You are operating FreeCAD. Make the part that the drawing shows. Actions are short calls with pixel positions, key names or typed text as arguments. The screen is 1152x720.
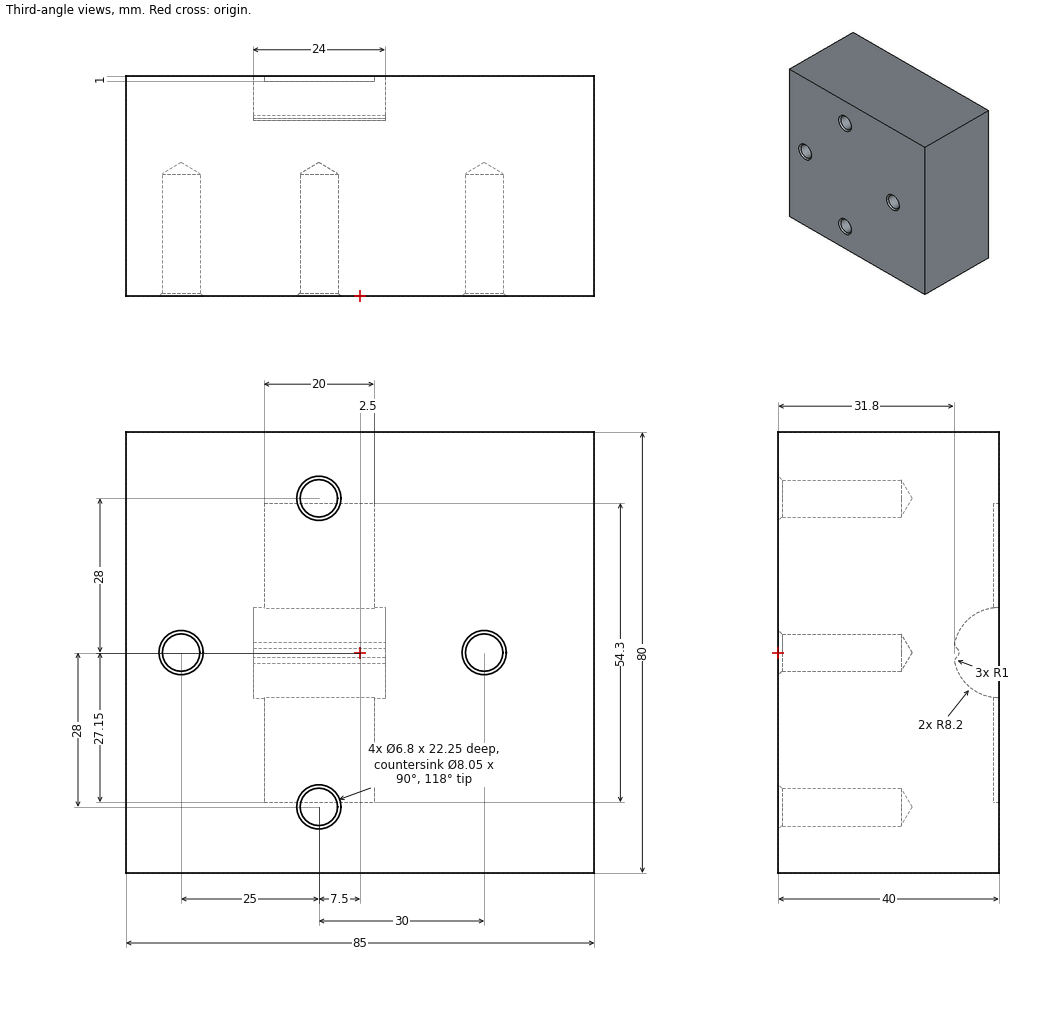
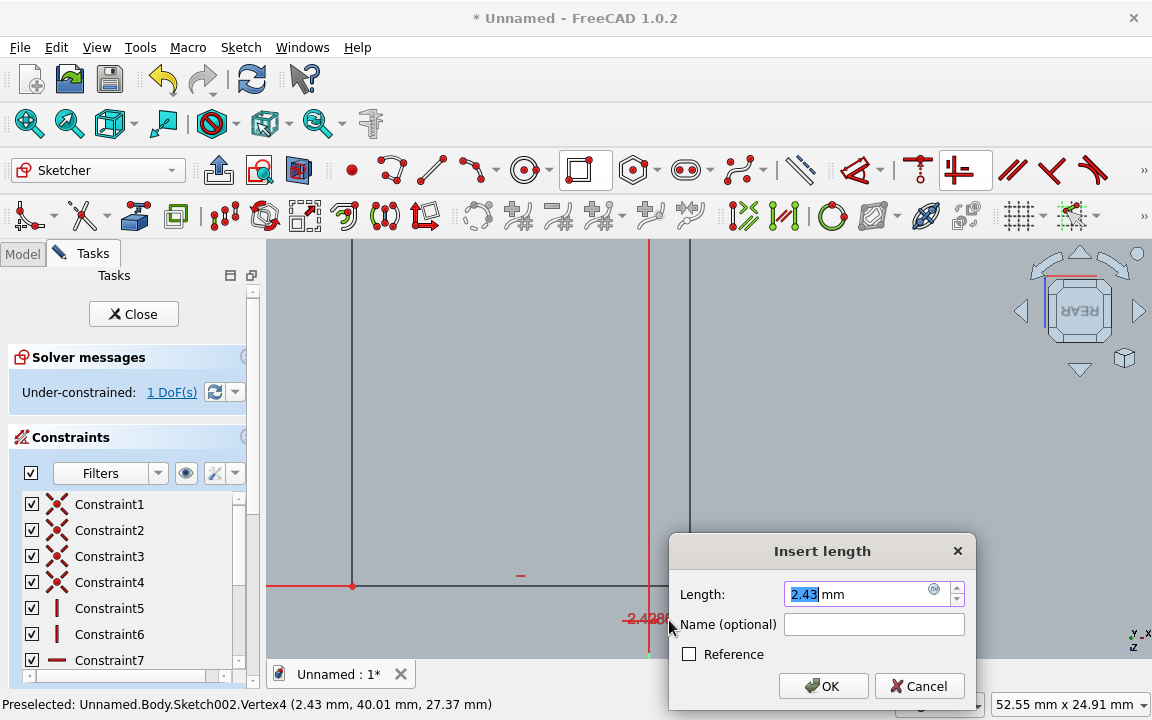
text(2.5)
key(Return)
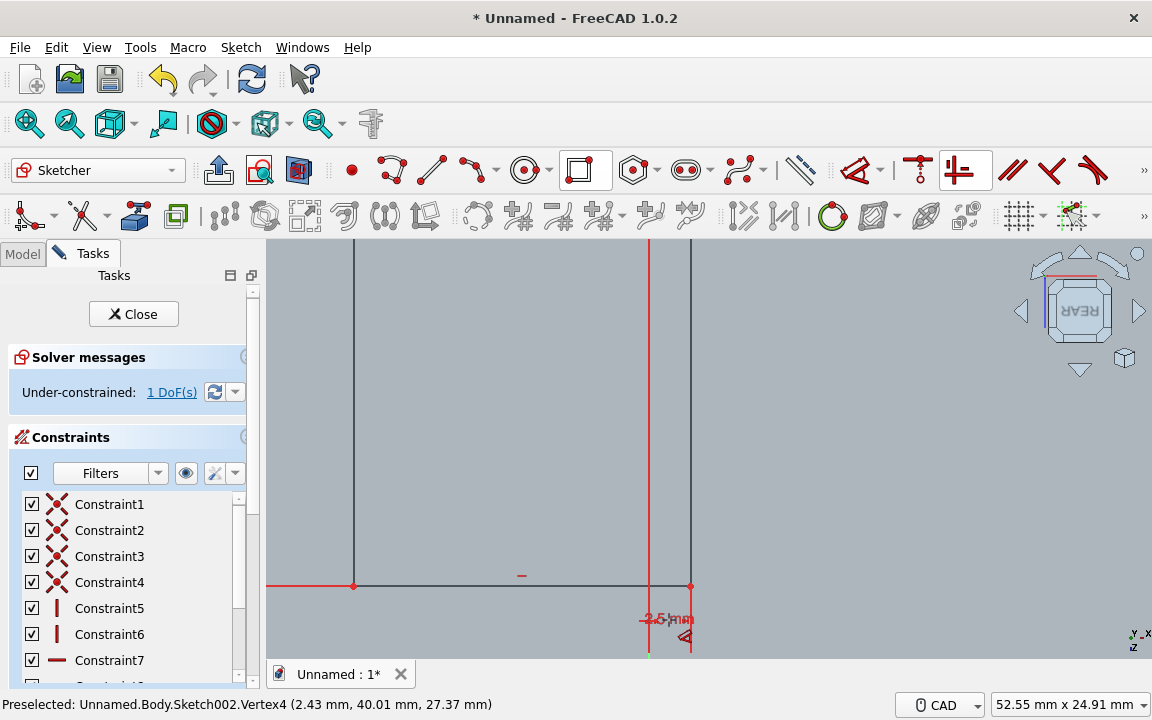
scroll(691, 589, down, 6)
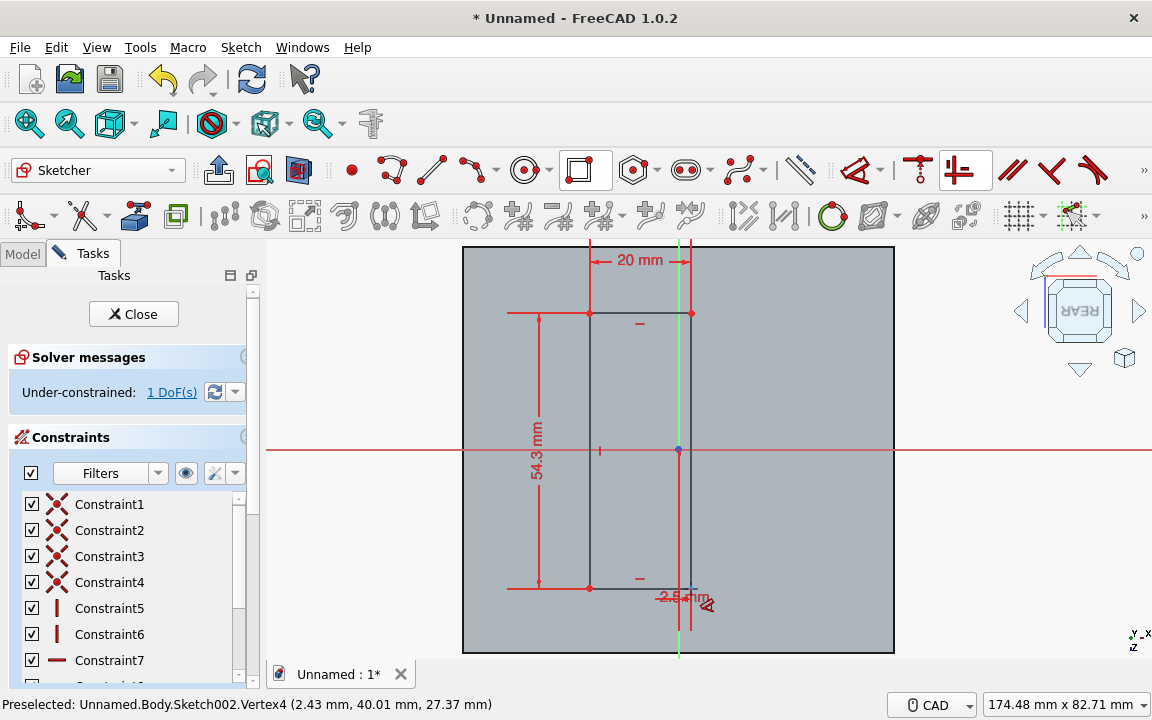
click(590, 313)
click(556, 381)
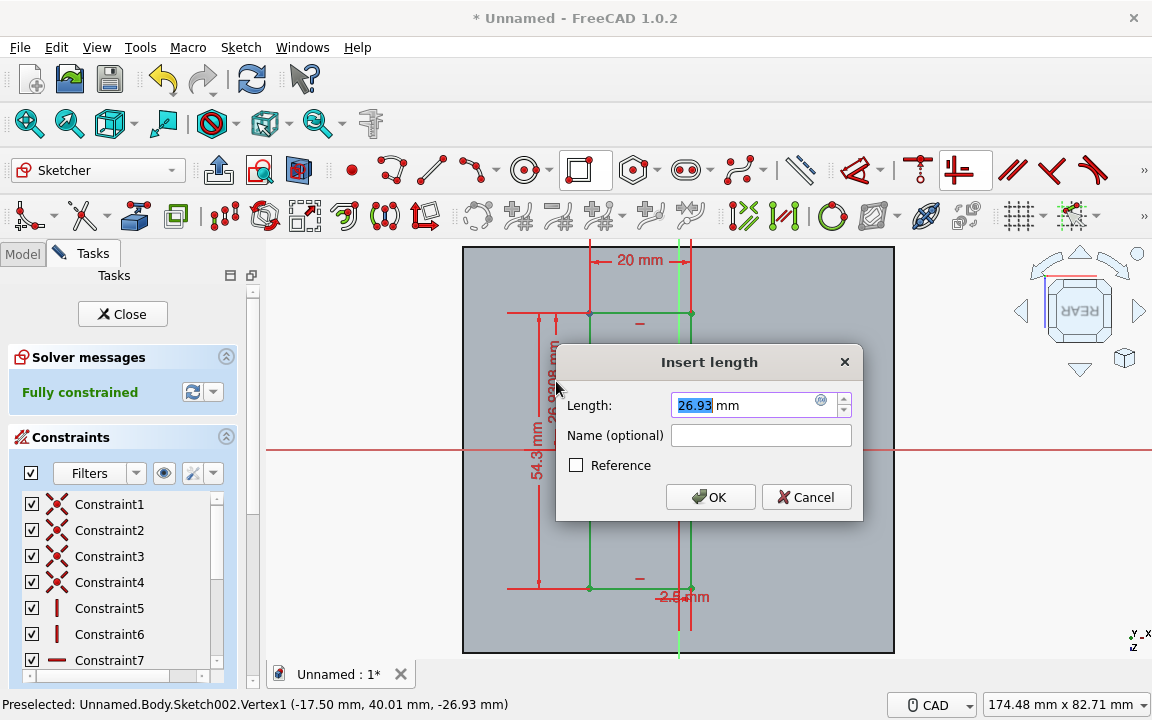
text(27.15)
key(Return)
key(Escape)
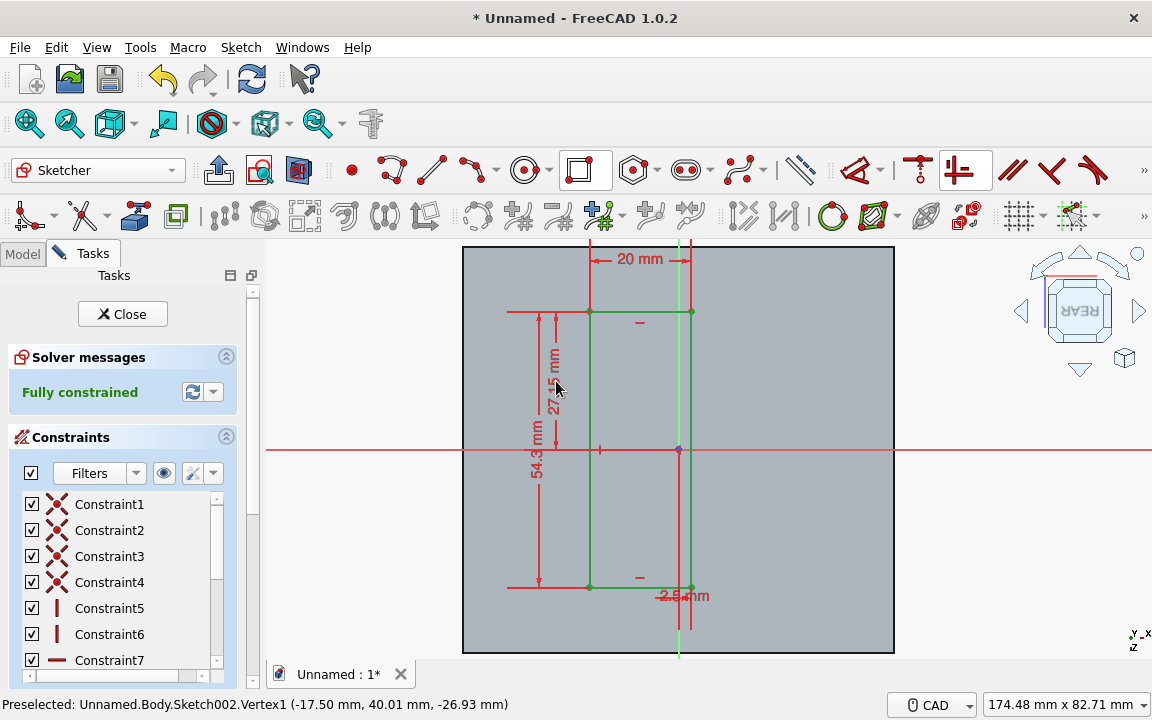
click(123, 314)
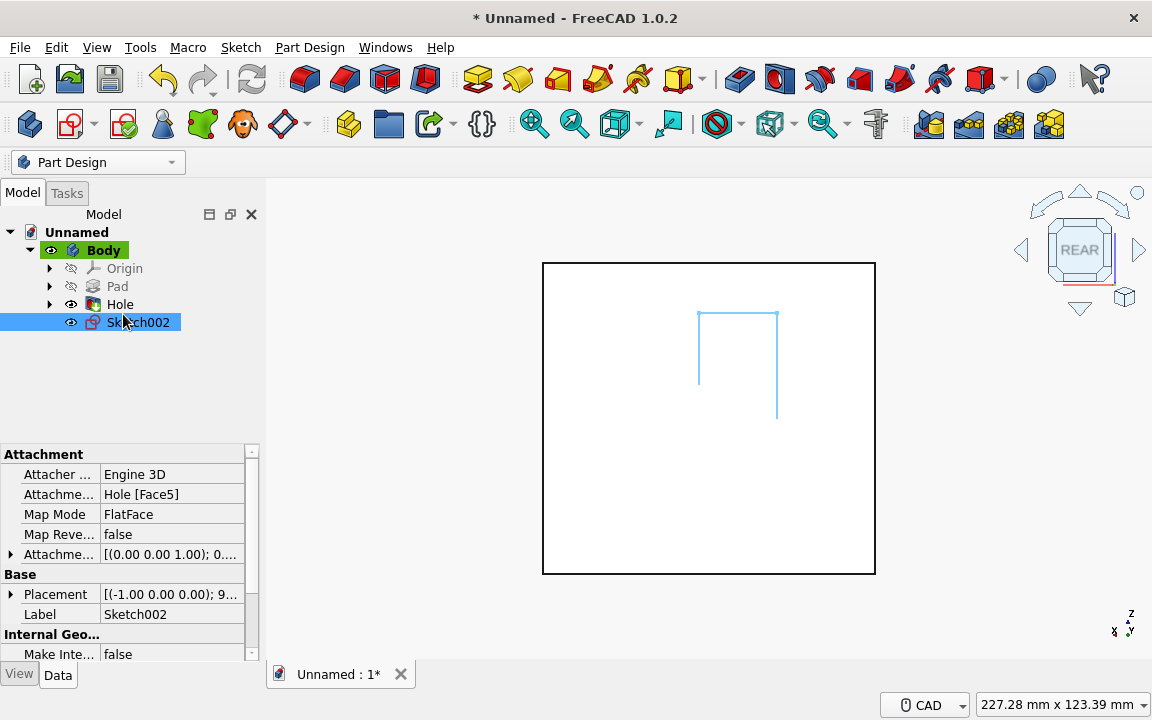
click(740, 80)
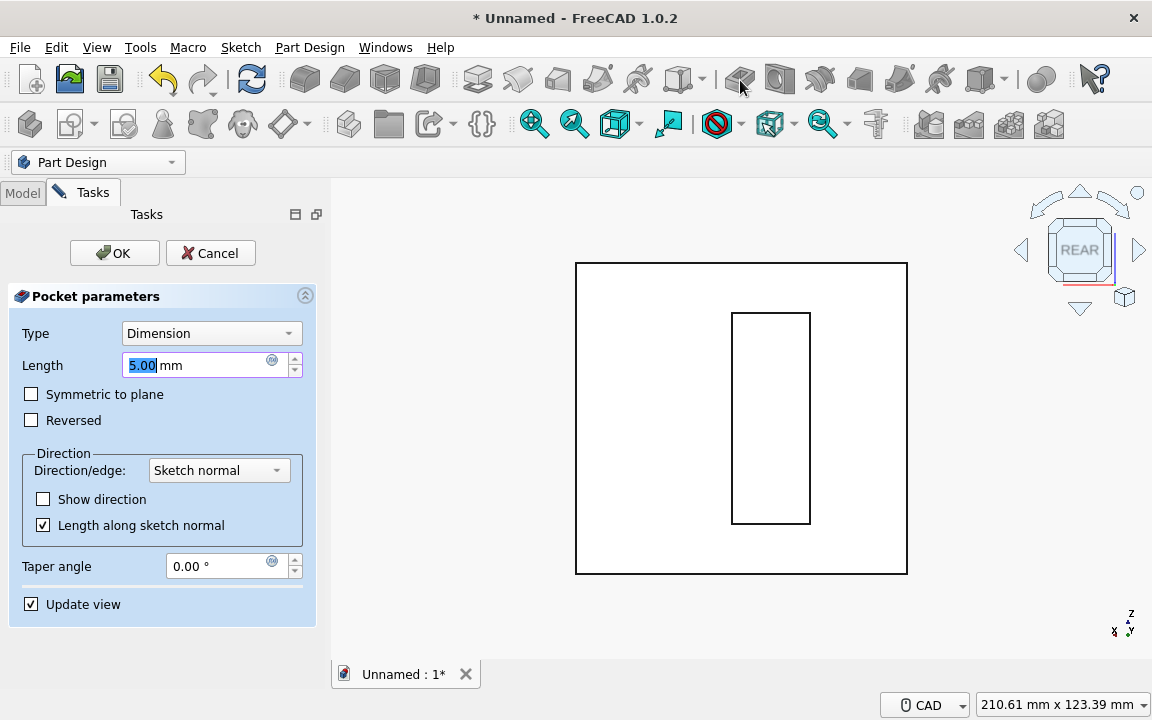
text(1)
key(Tab)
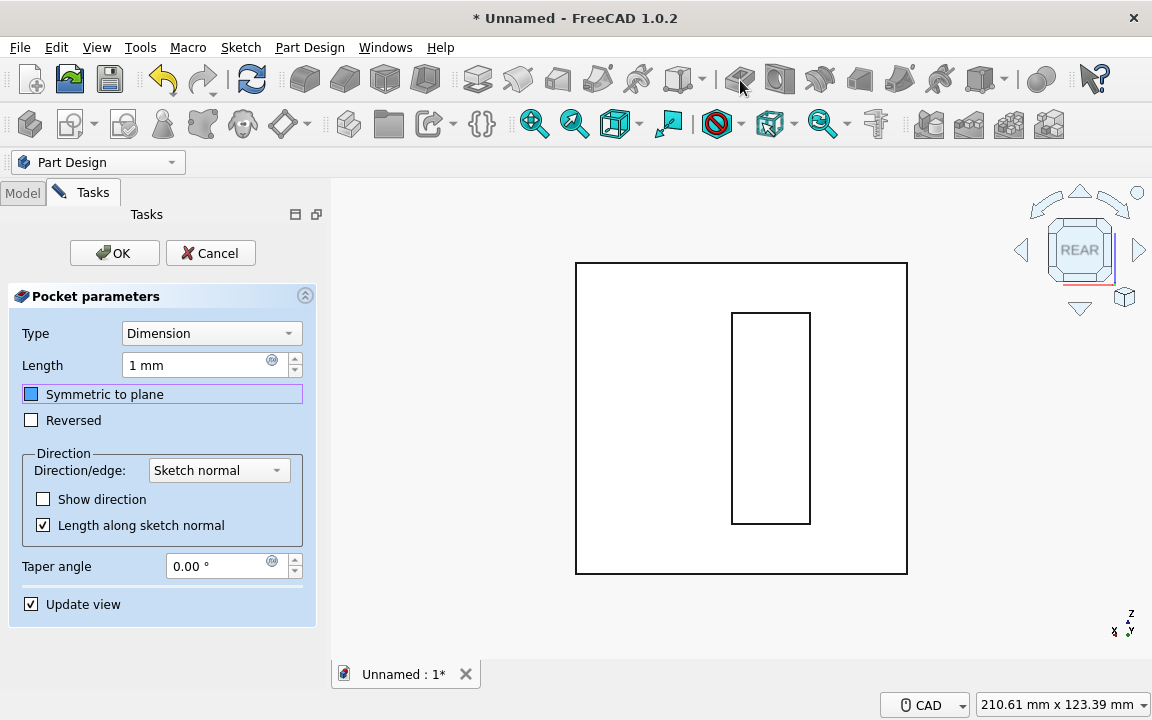
click(115, 253)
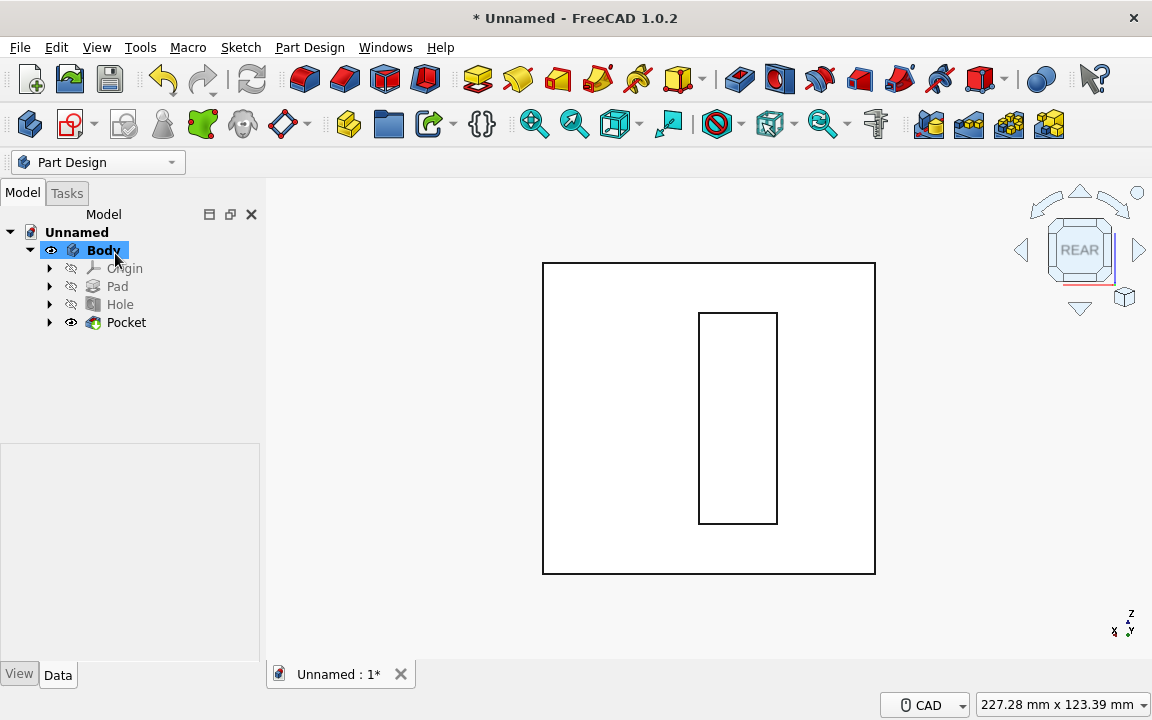
click(50, 268)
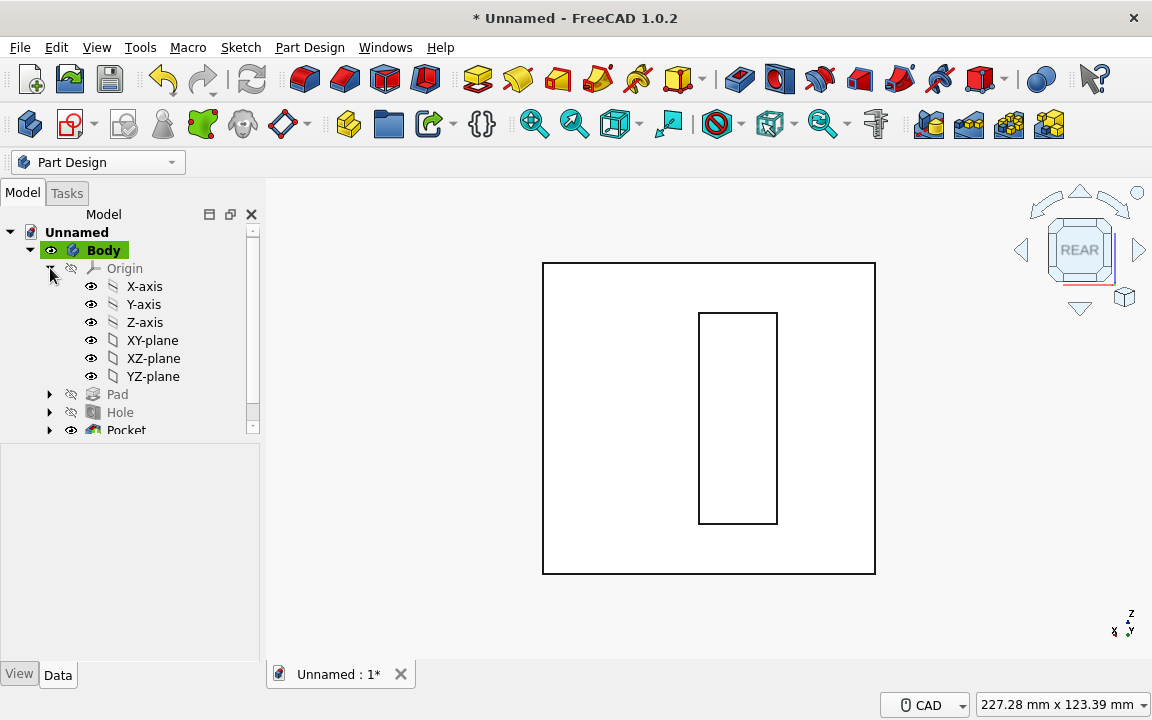
click(136, 376)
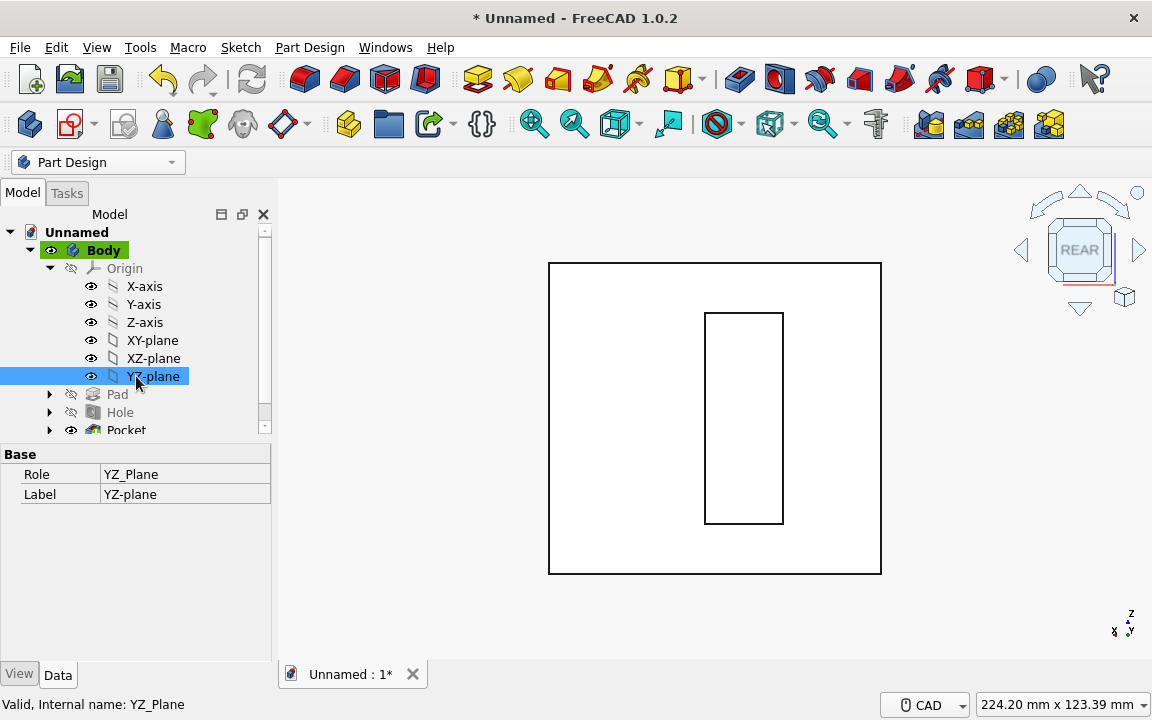
click(284, 124)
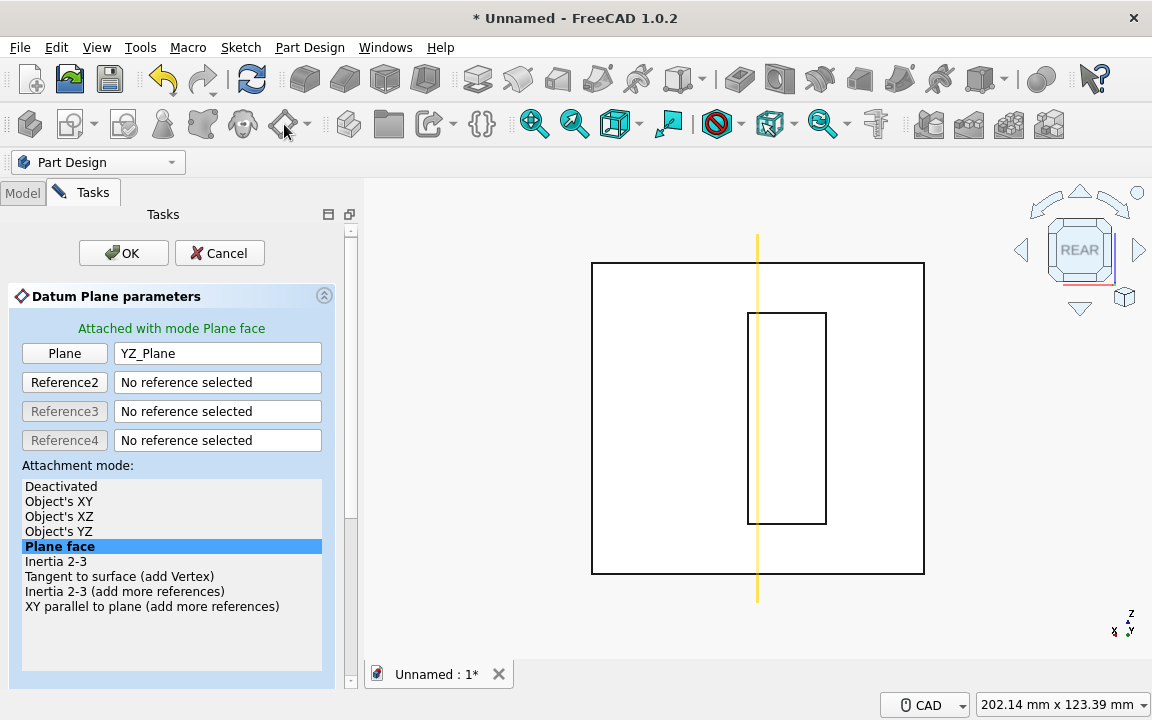
scroll(351, 456, down, 3)